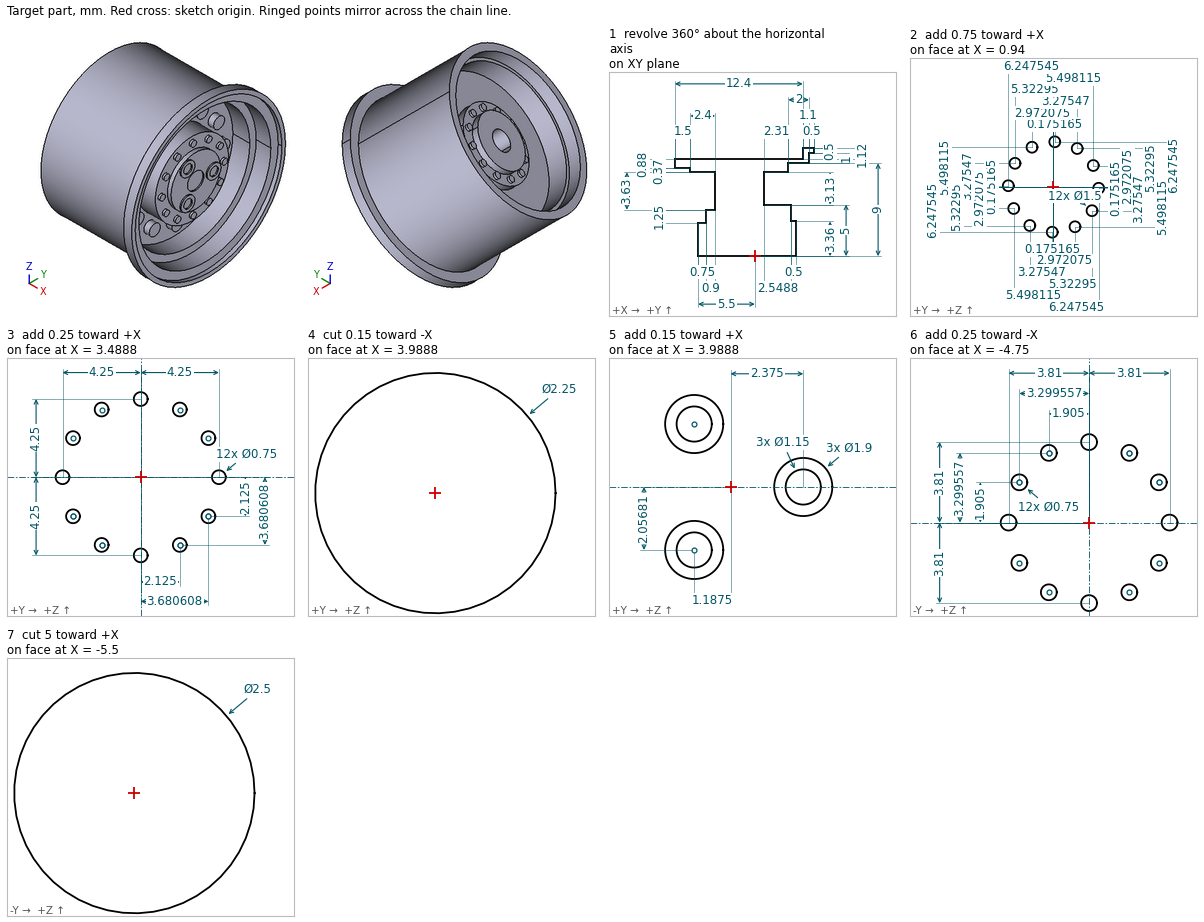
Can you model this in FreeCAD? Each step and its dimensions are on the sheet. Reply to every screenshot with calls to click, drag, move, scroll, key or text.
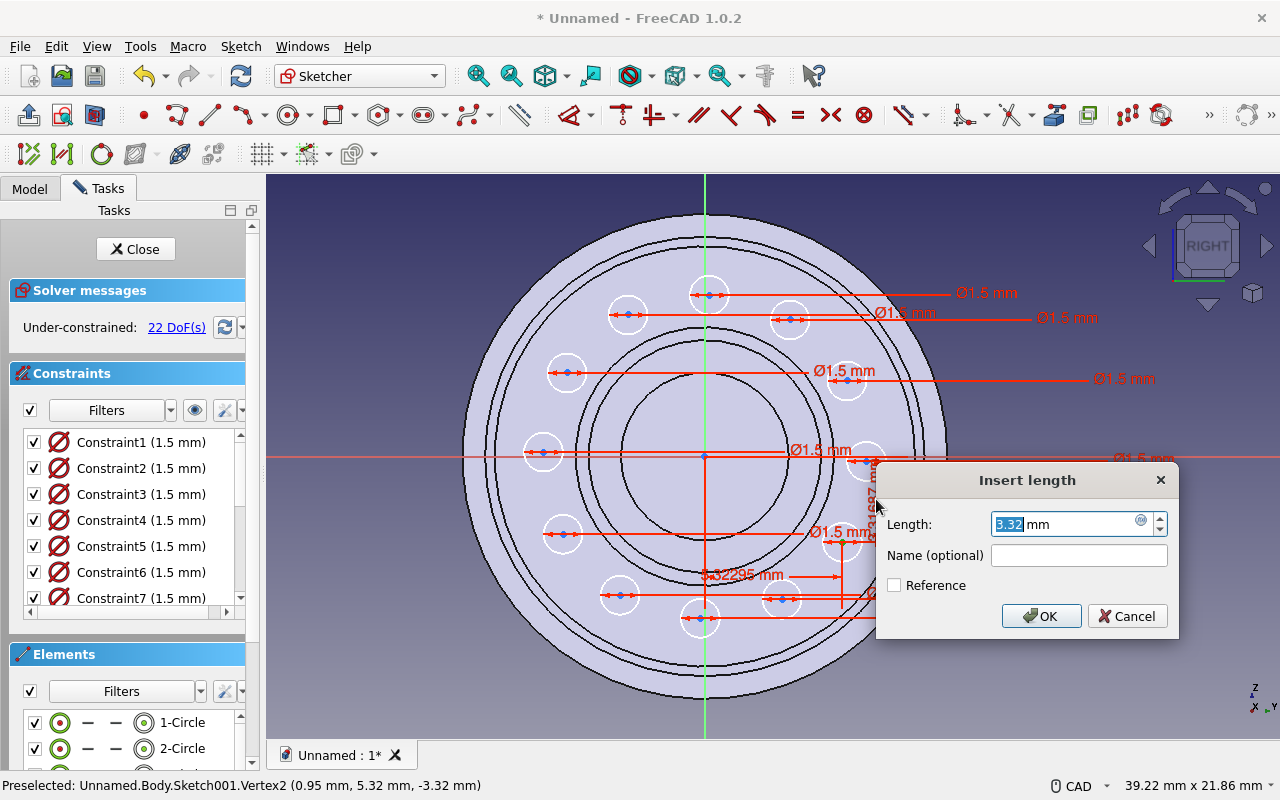
text(3.27547)
key(Return)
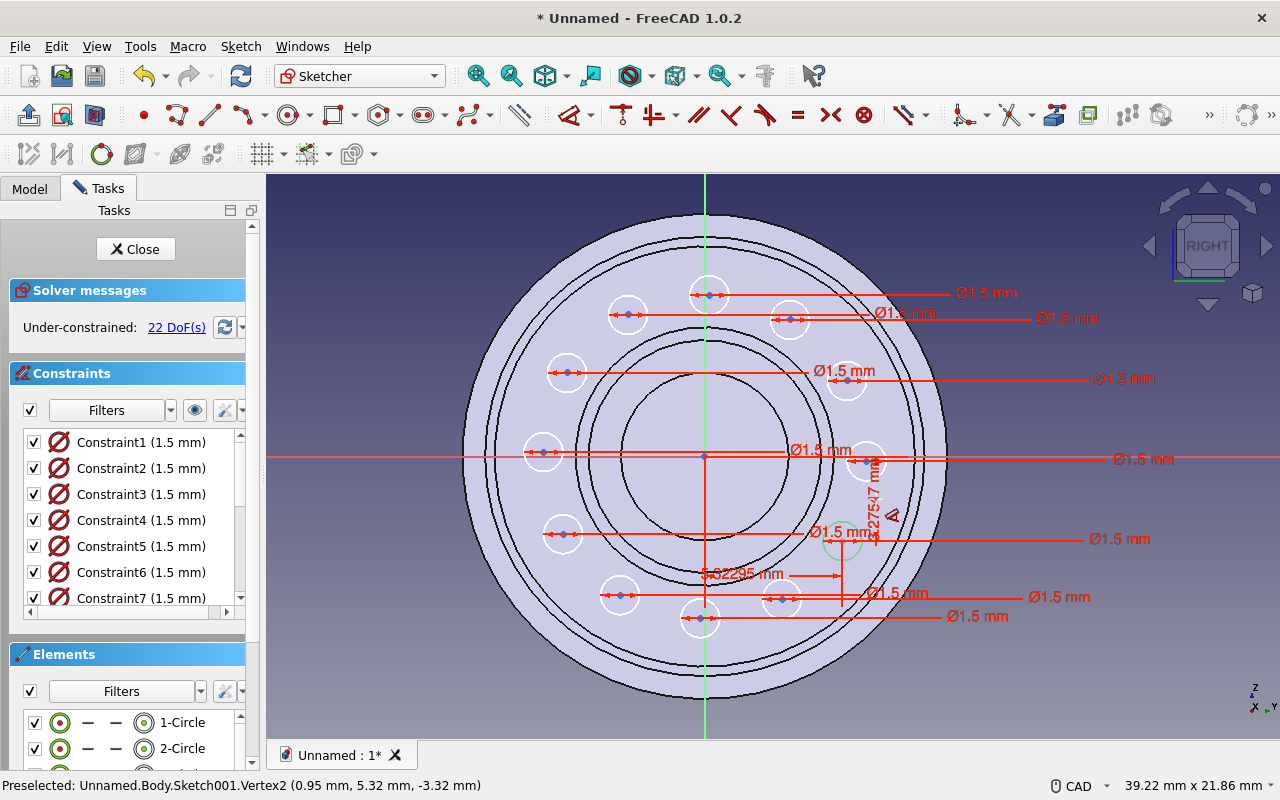
click(620, 595)
click(662, 629)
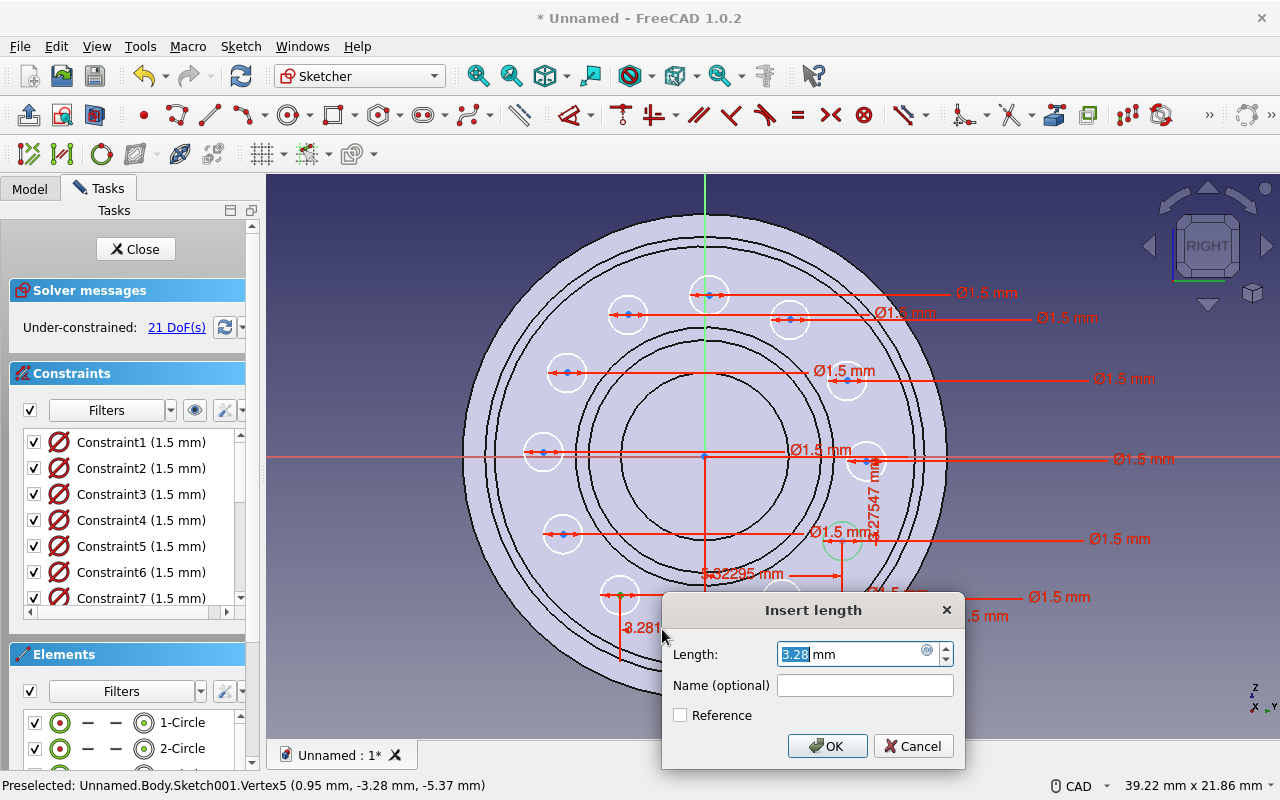
text(3.27547)
key(Return)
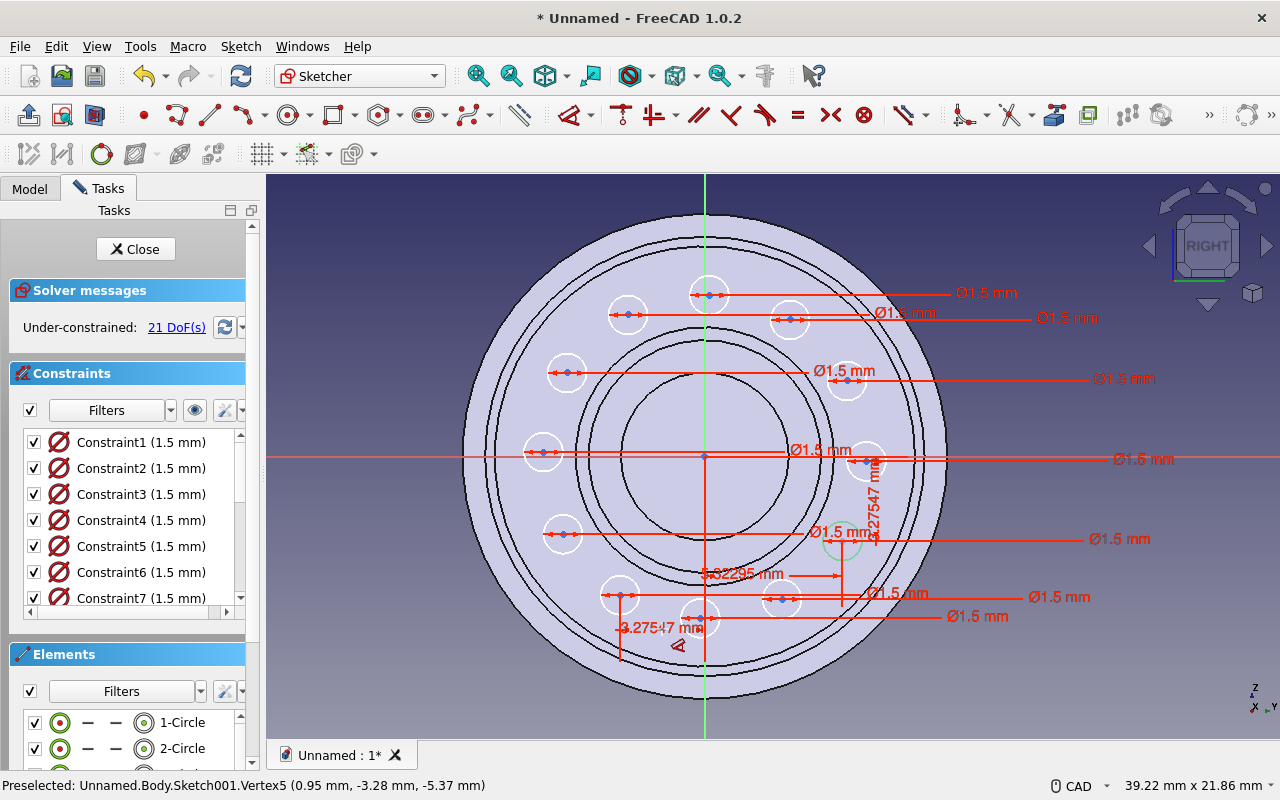
click(620, 595)
click(586, 494)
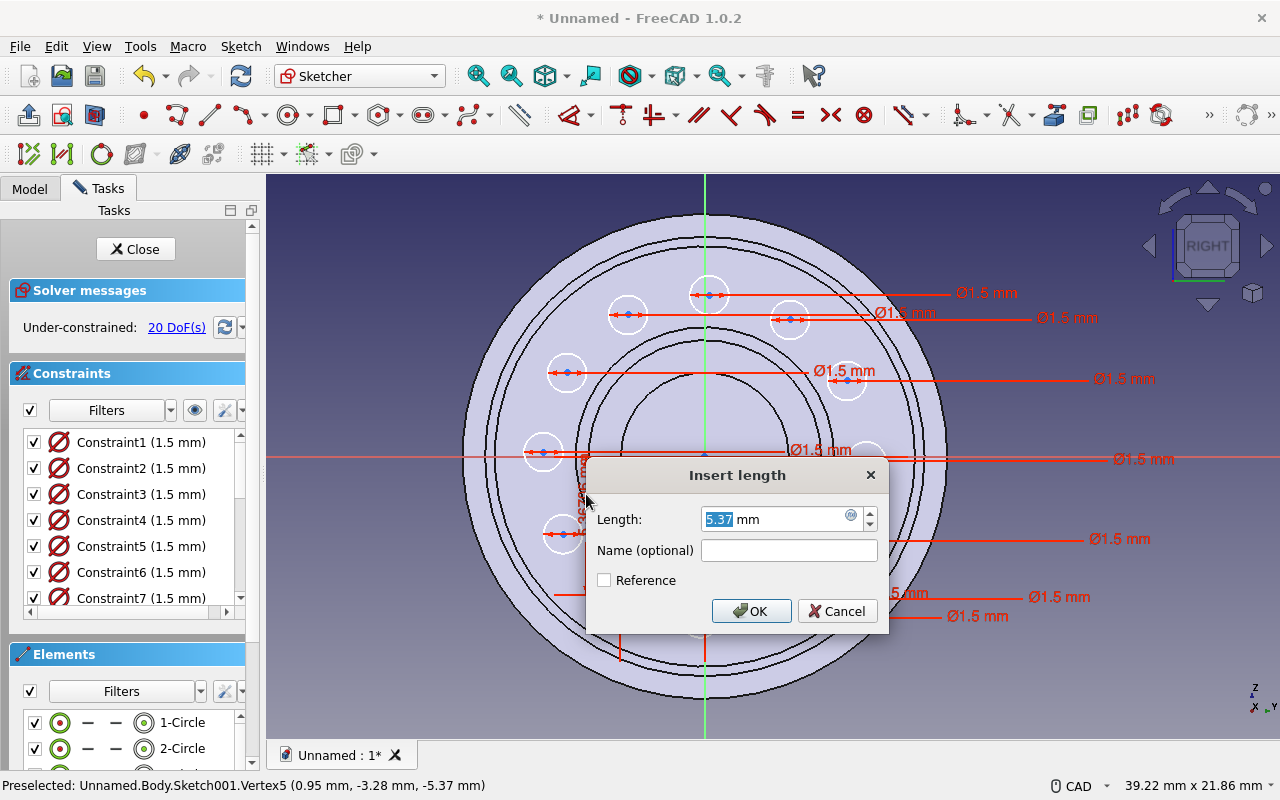
text(5.32295)
key(Return)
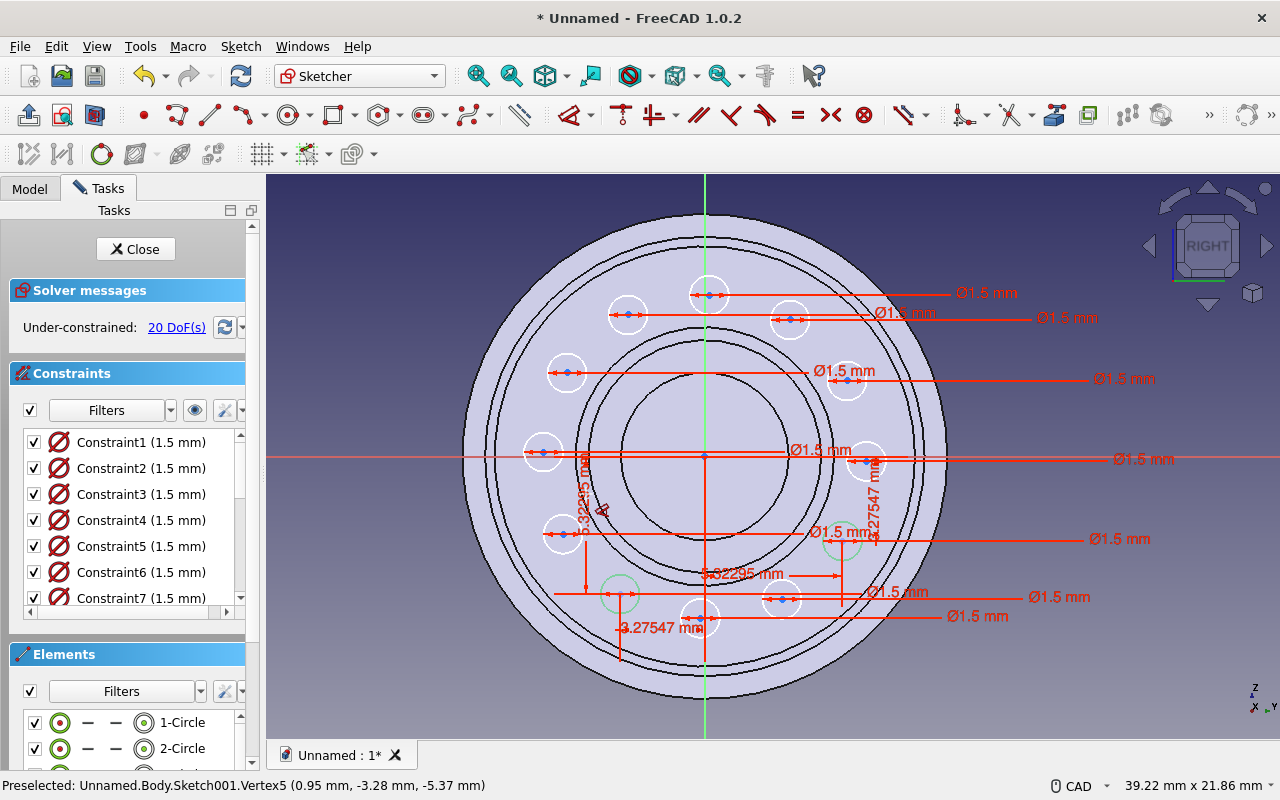
click(567, 373)
click(604, 339)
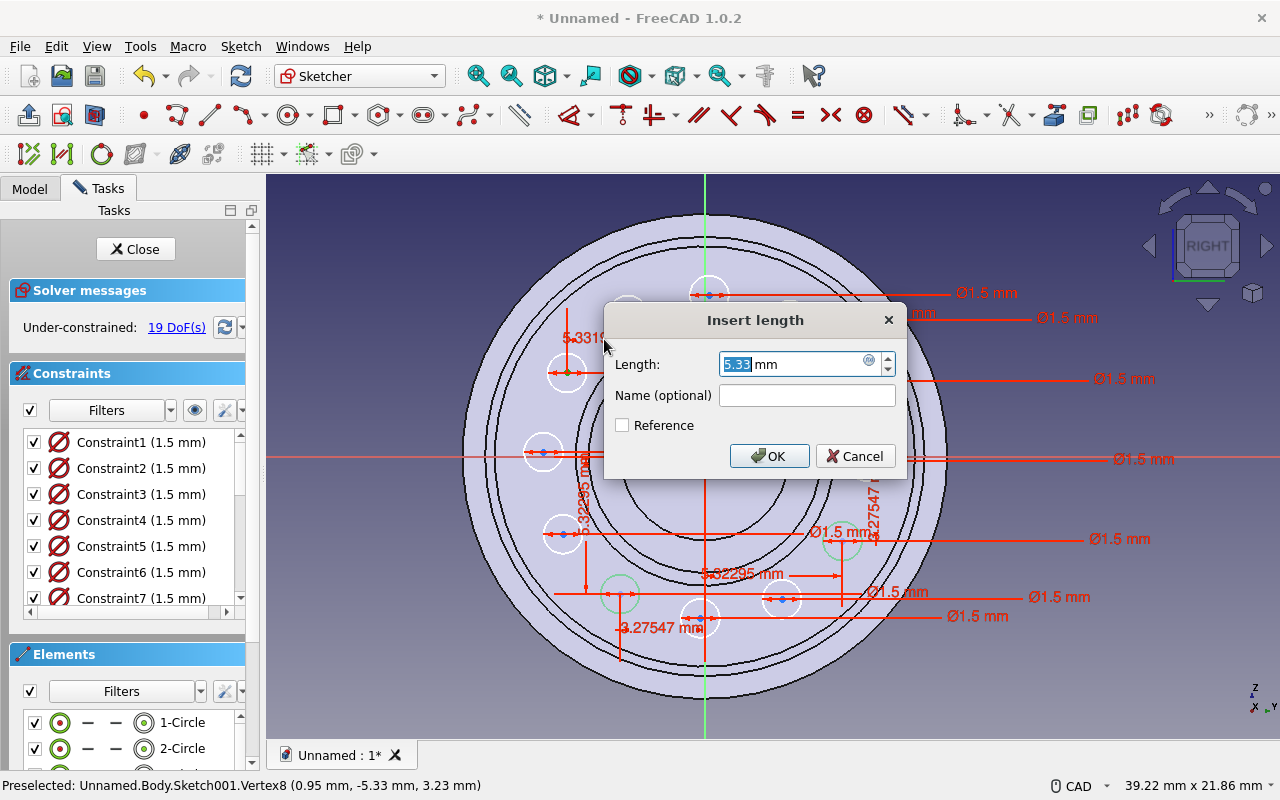
text(5.32295)
key(Return)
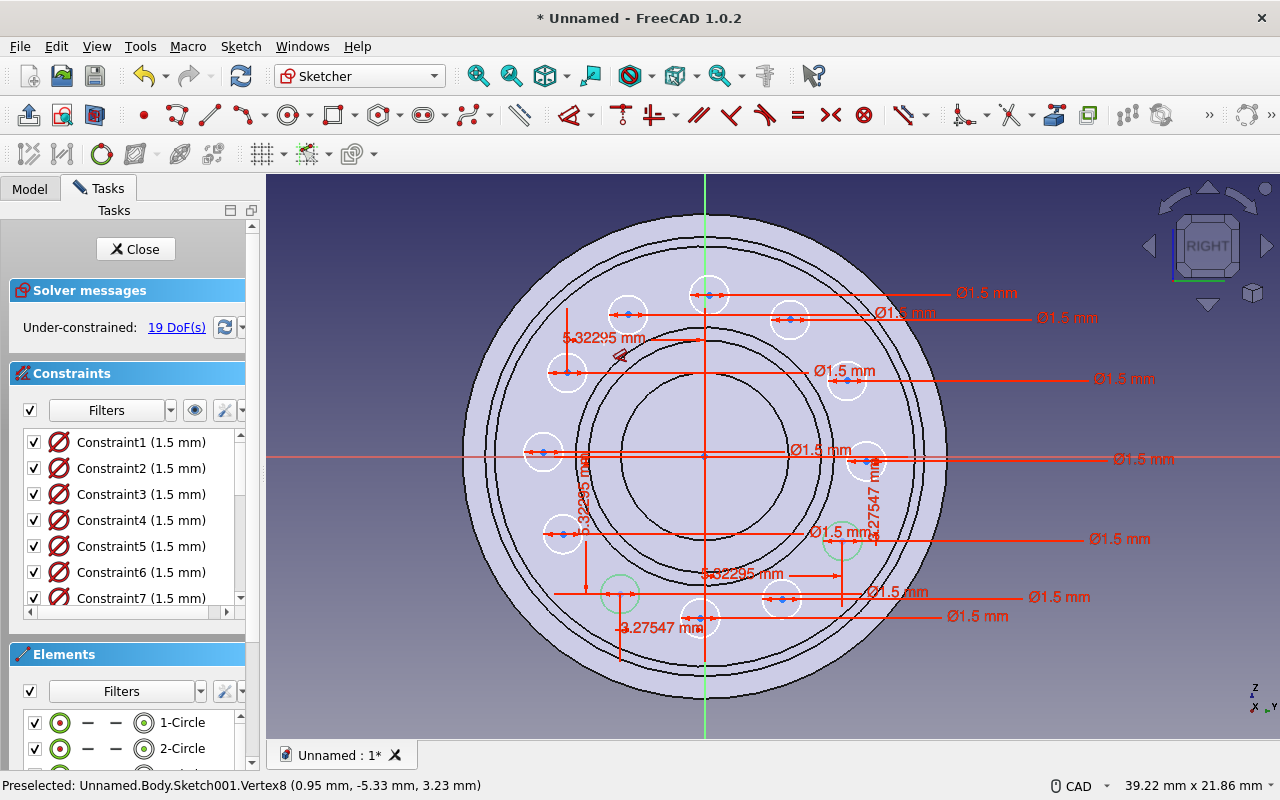
click(567, 373)
click(533, 415)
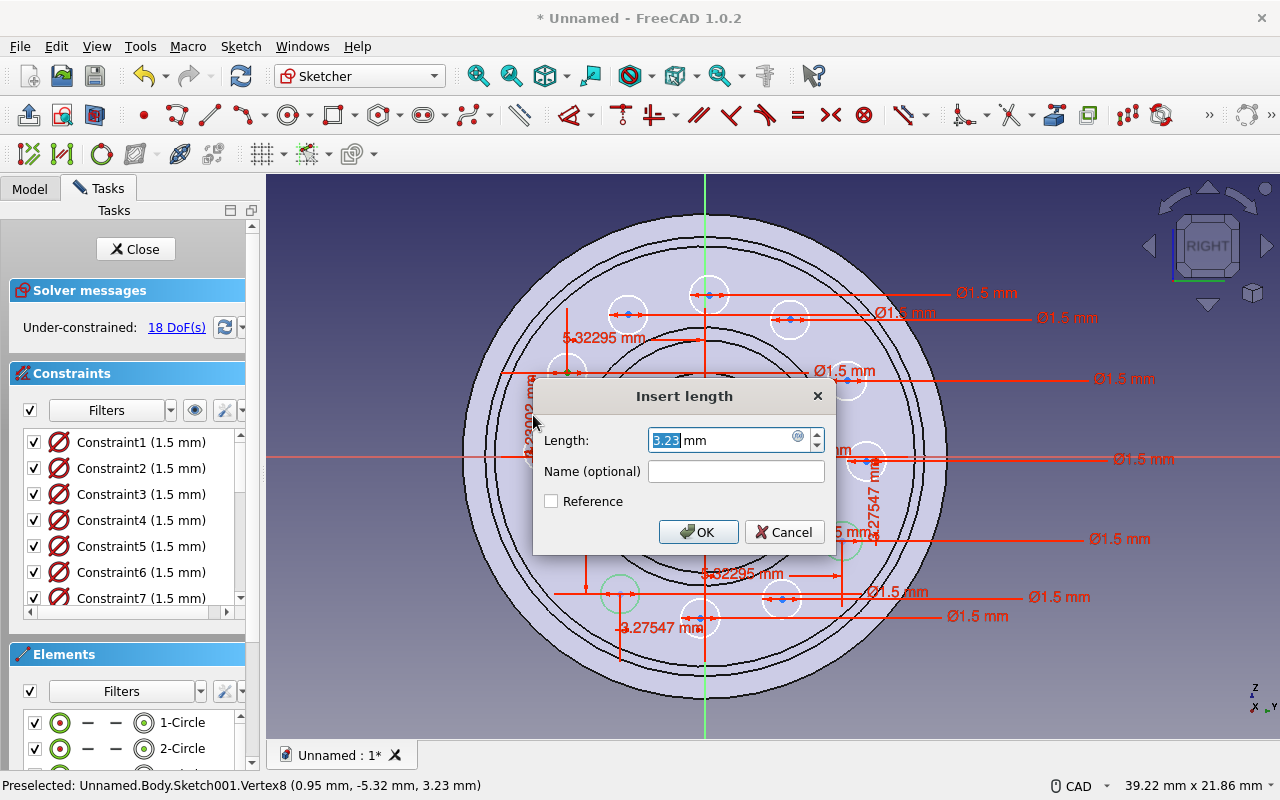
text(3.27547)
key(Return)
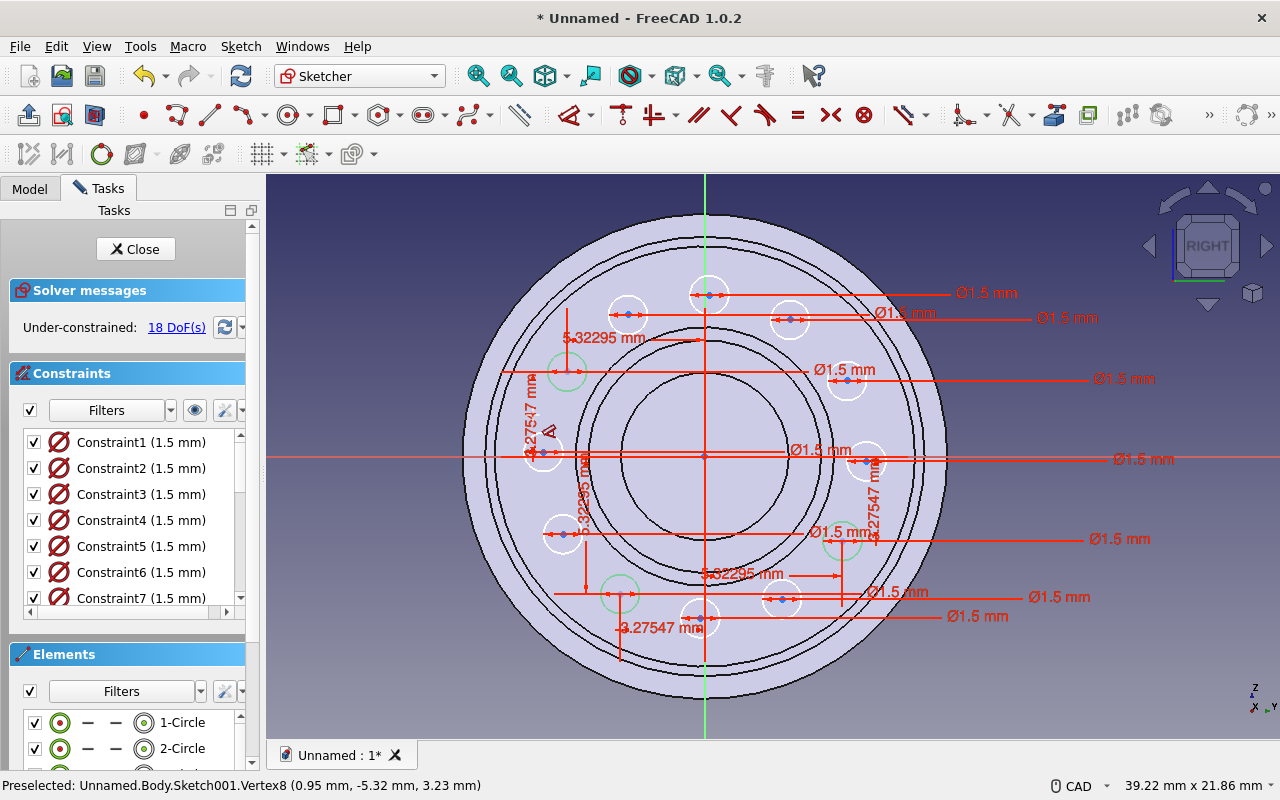
click(790, 320)
click(747, 286)